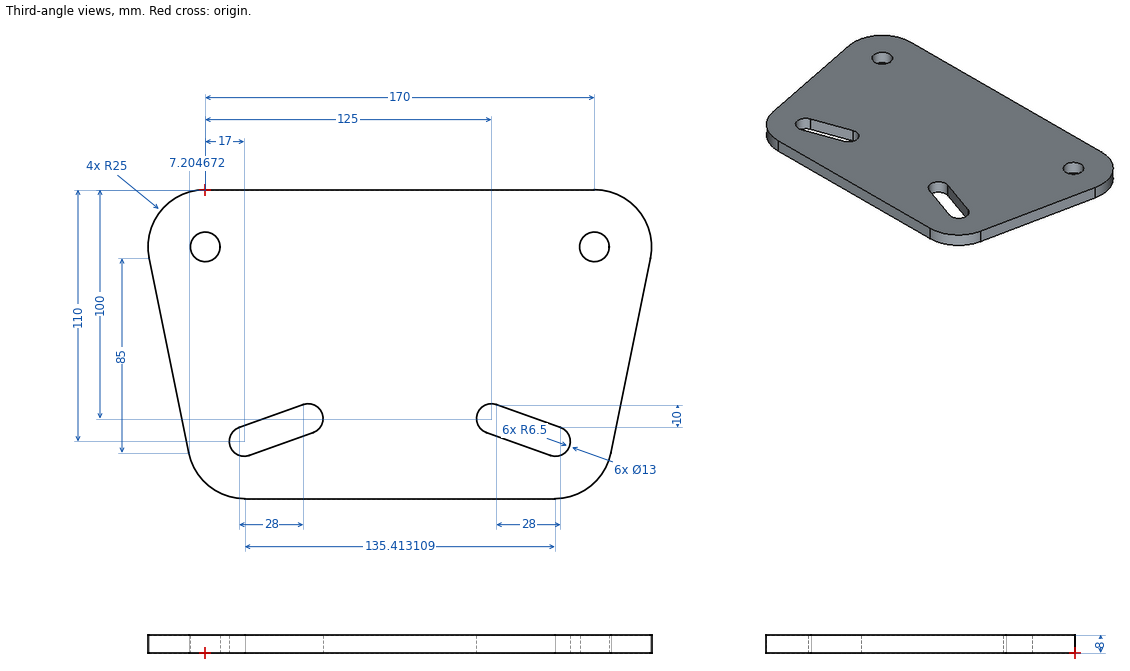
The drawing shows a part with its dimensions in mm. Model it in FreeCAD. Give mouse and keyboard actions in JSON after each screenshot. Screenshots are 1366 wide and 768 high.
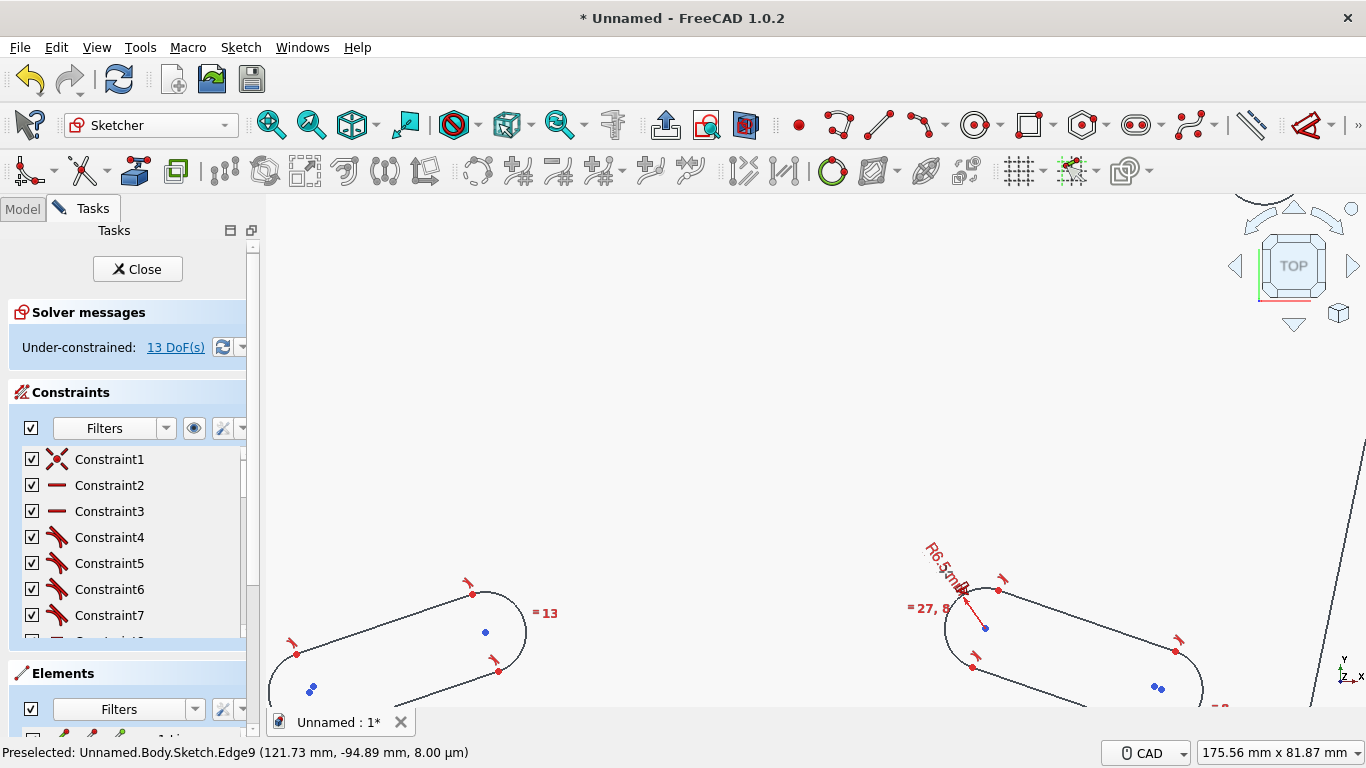
{"action": "scroll", "coordinate": [754, 465], "scroll_direction": "down", "scroll_amount": 5}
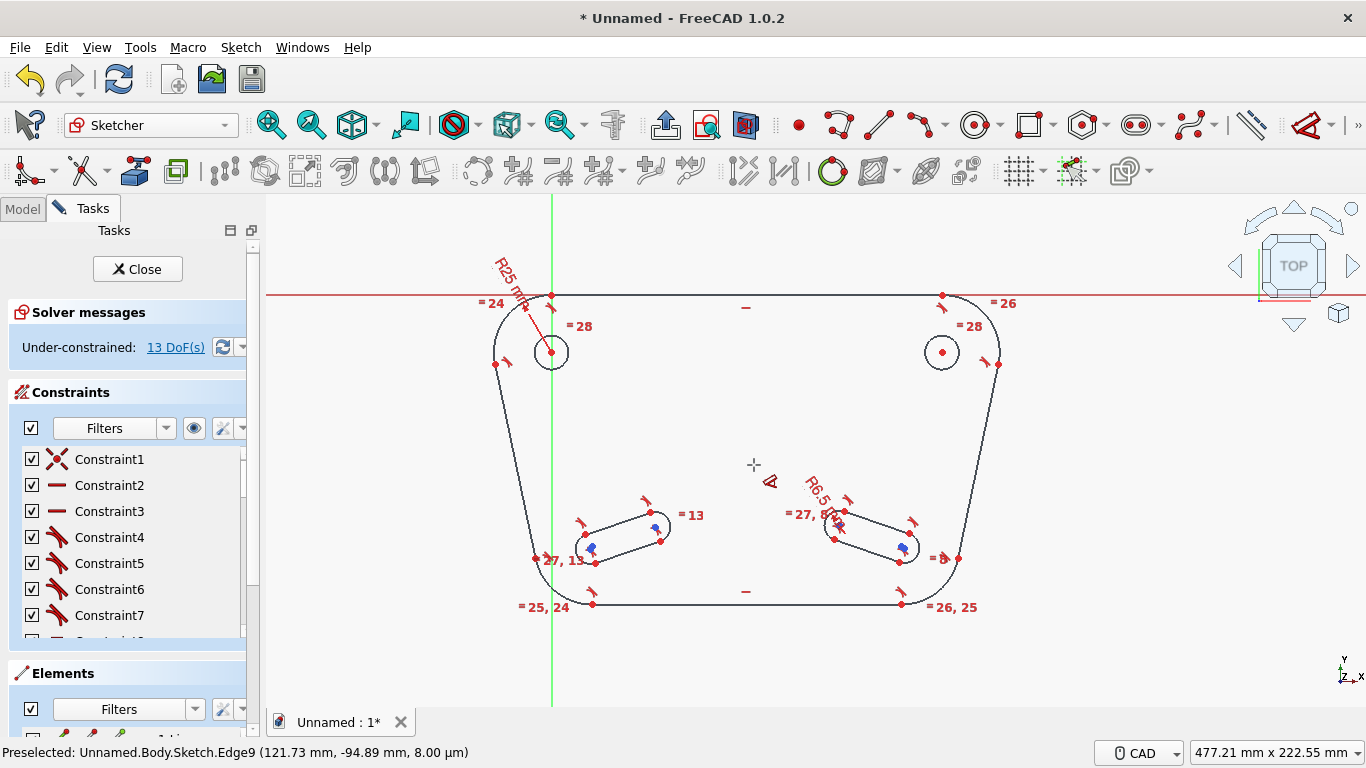
{"action": "scroll", "coordinate": [954, 341], "scroll_direction": "up", "scroll_amount": 2}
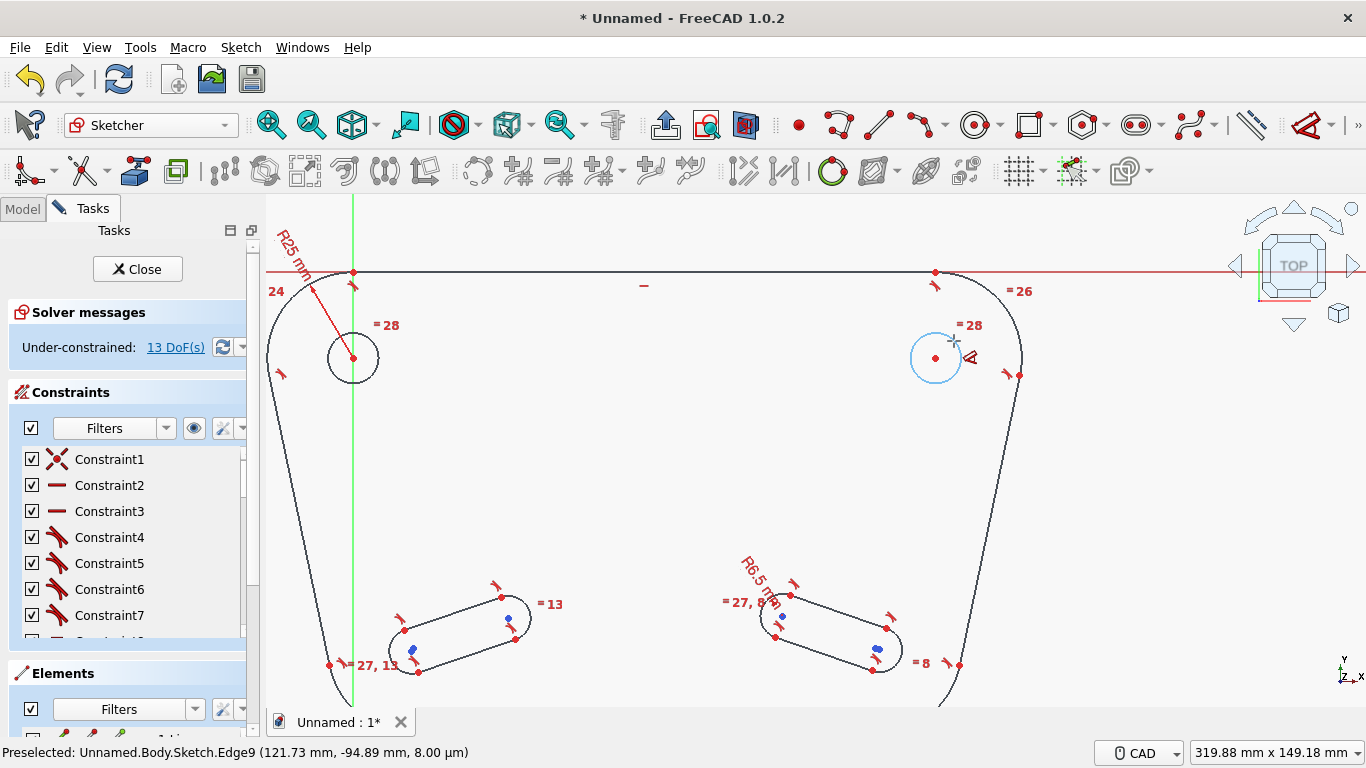
{"action": "left_click", "coordinate": [954, 340]}
{"action": "left_click", "coordinate": [977, 317]}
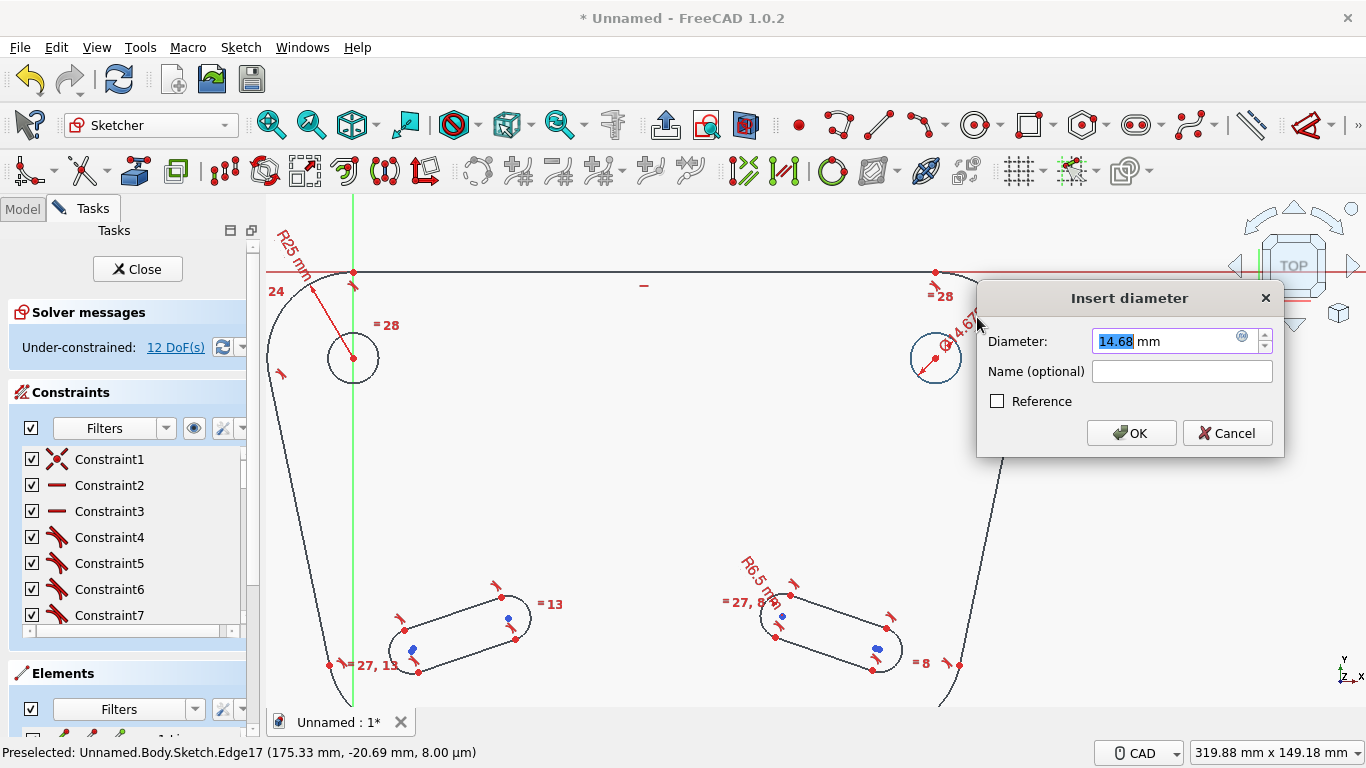
{"action": "type", "text": "13"}
{"action": "key", "text": "Return"}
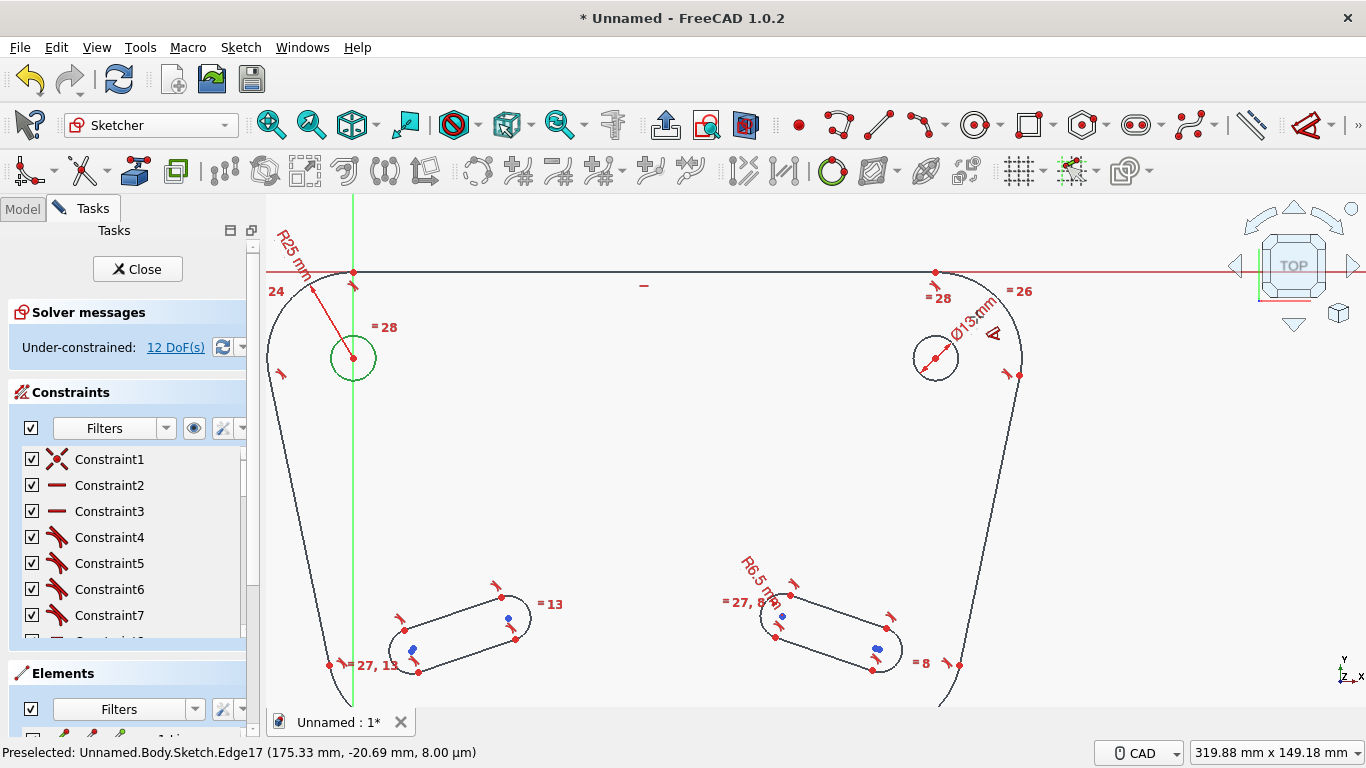
{"action": "left_click", "coordinate": [761, 272]}
{"action": "left_click", "coordinate": [645, 238]}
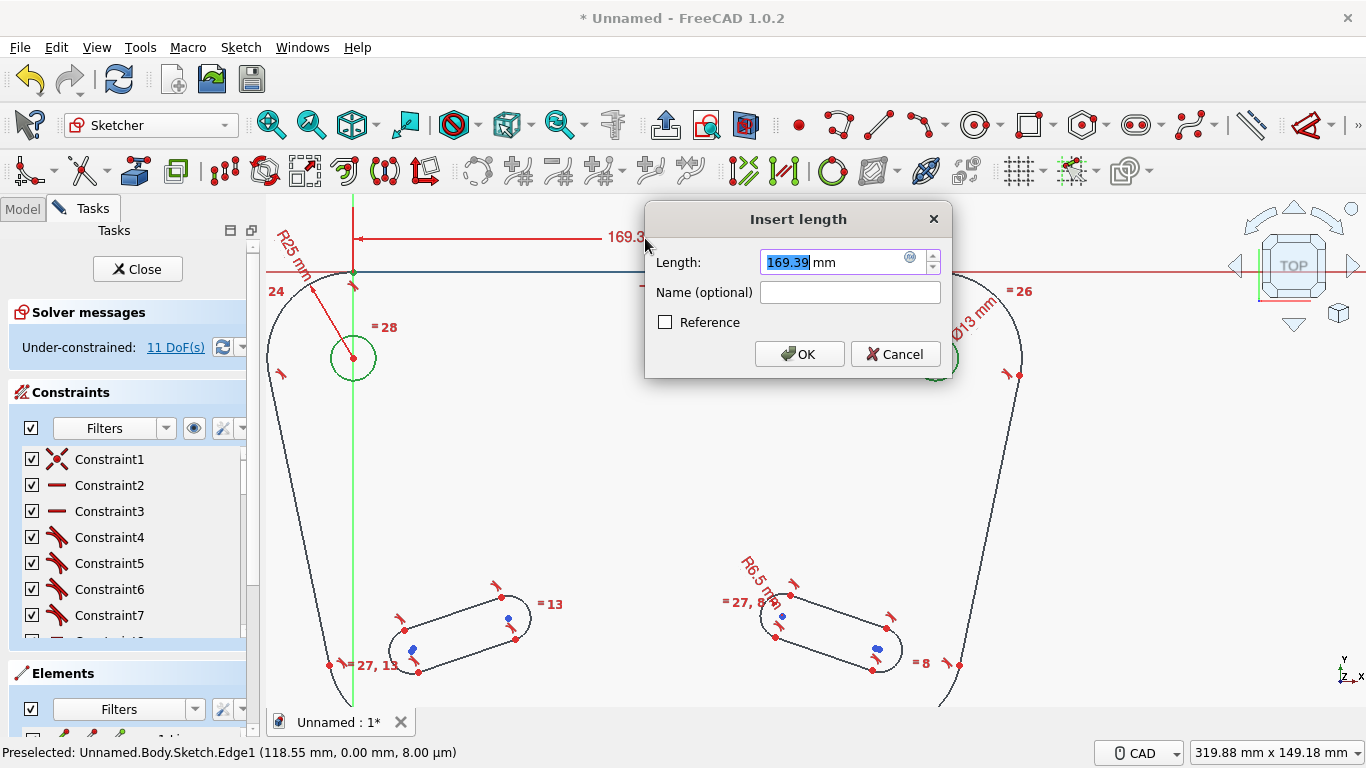
{"action": "type", "text": "170"}
{"action": "key", "text": "Return"}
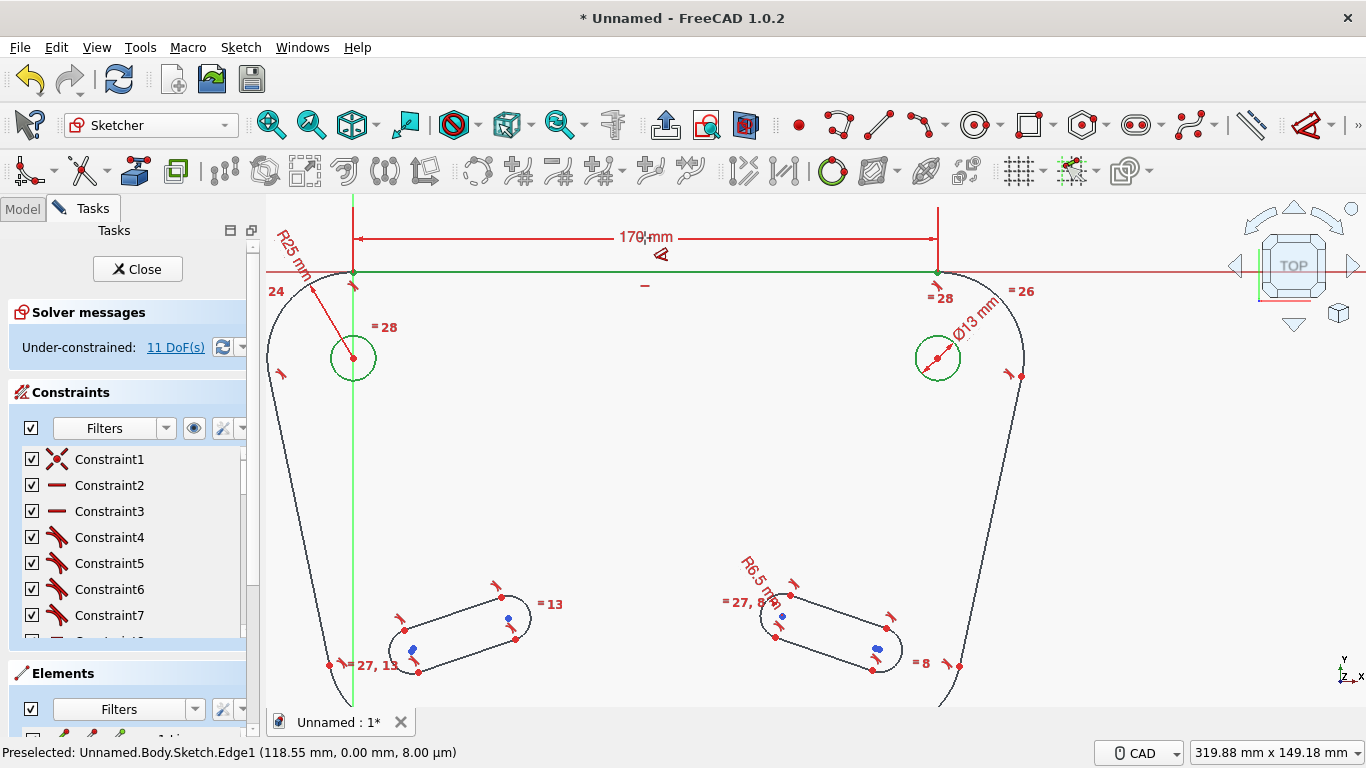
{"action": "left_click", "coordinate": [311, 579]}
{"action": "left_click", "coordinate": [388, 521]}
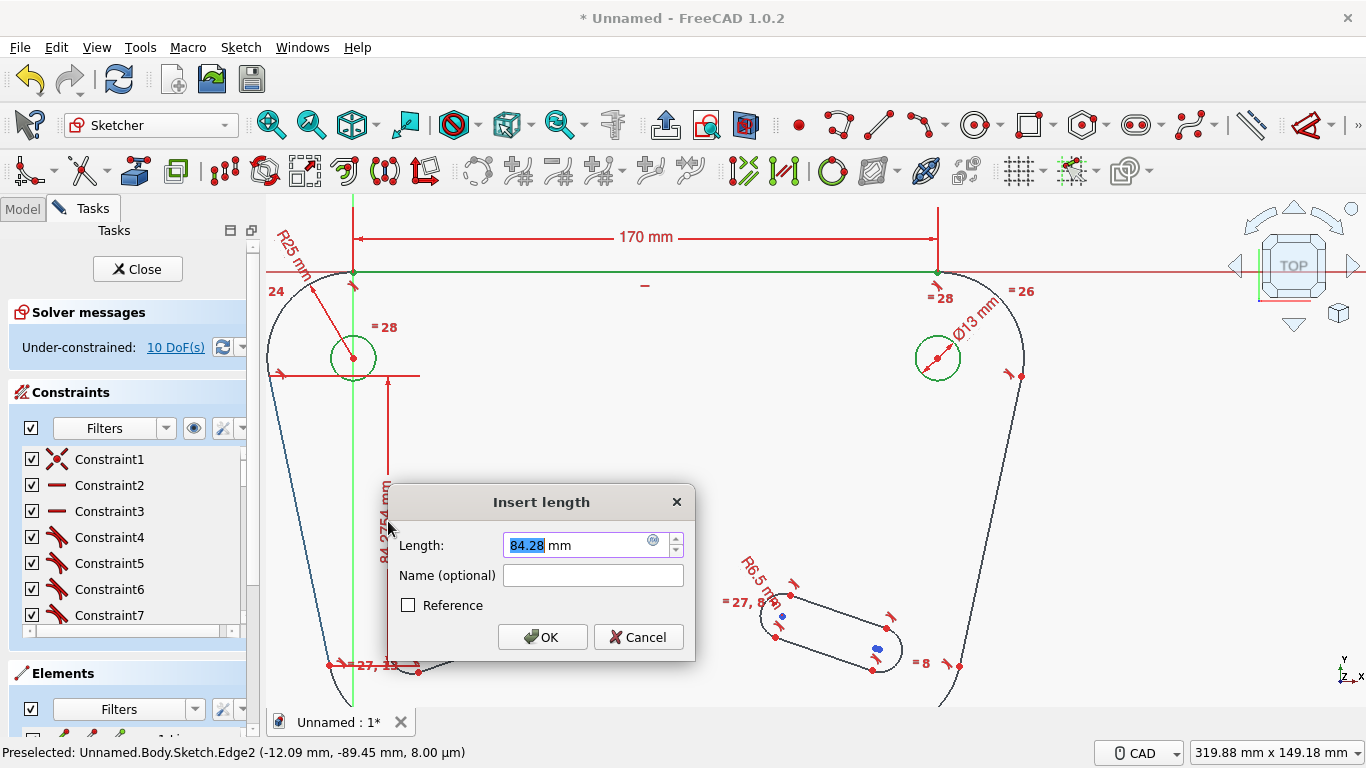
{"action": "type", "text": "85"}
{"action": "key", "text": "Return"}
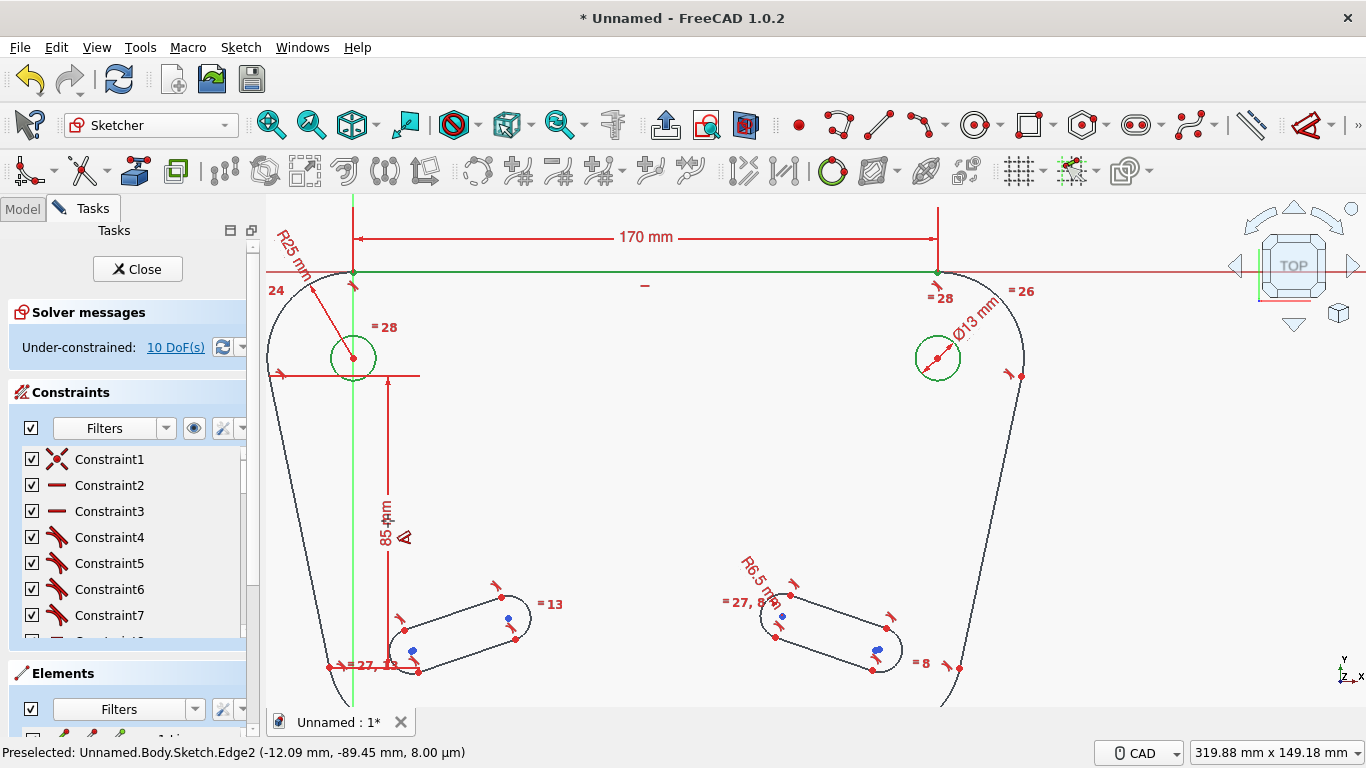
{"action": "left_click", "coordinate": [819, 605]}
{"action": "left_click", "coordinate": [805, 663]}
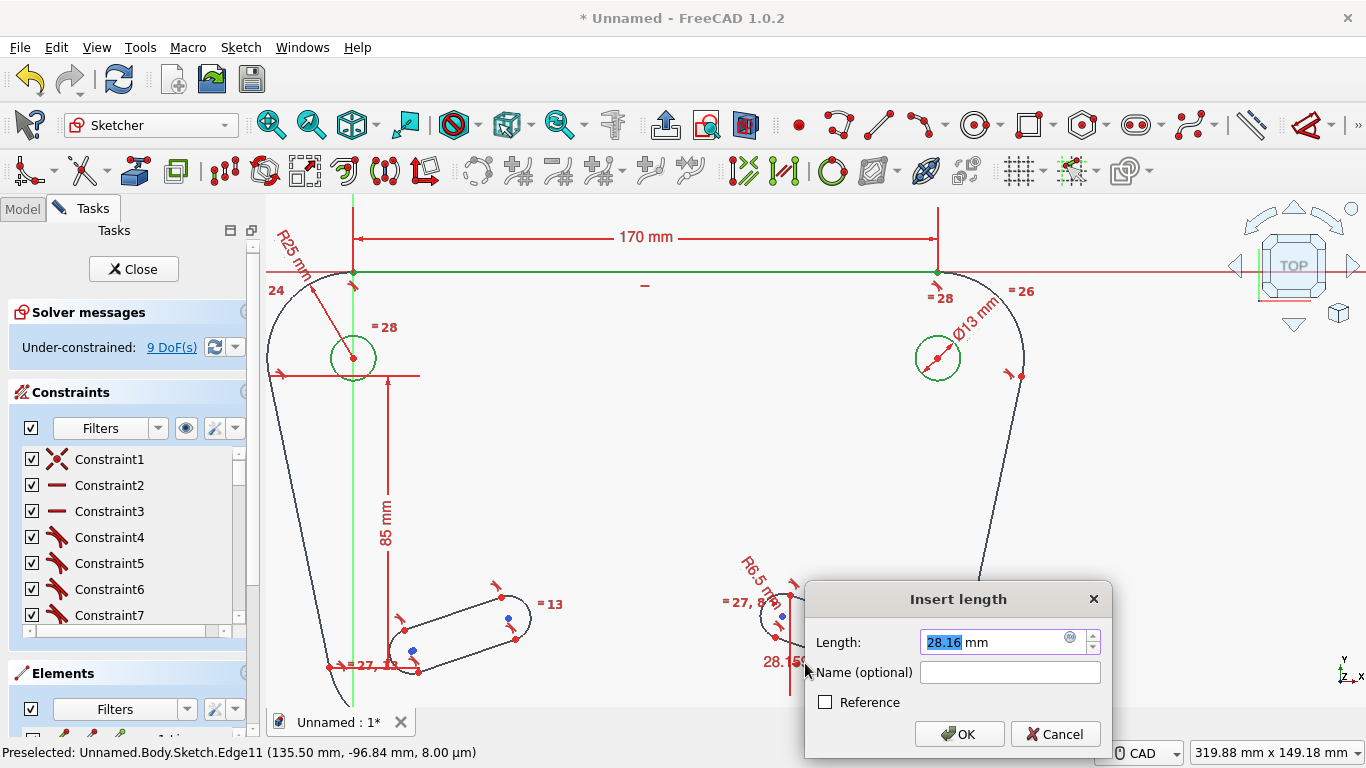
{"action": "type", "text": "28"}
{"action": "key", "text": "Return"}